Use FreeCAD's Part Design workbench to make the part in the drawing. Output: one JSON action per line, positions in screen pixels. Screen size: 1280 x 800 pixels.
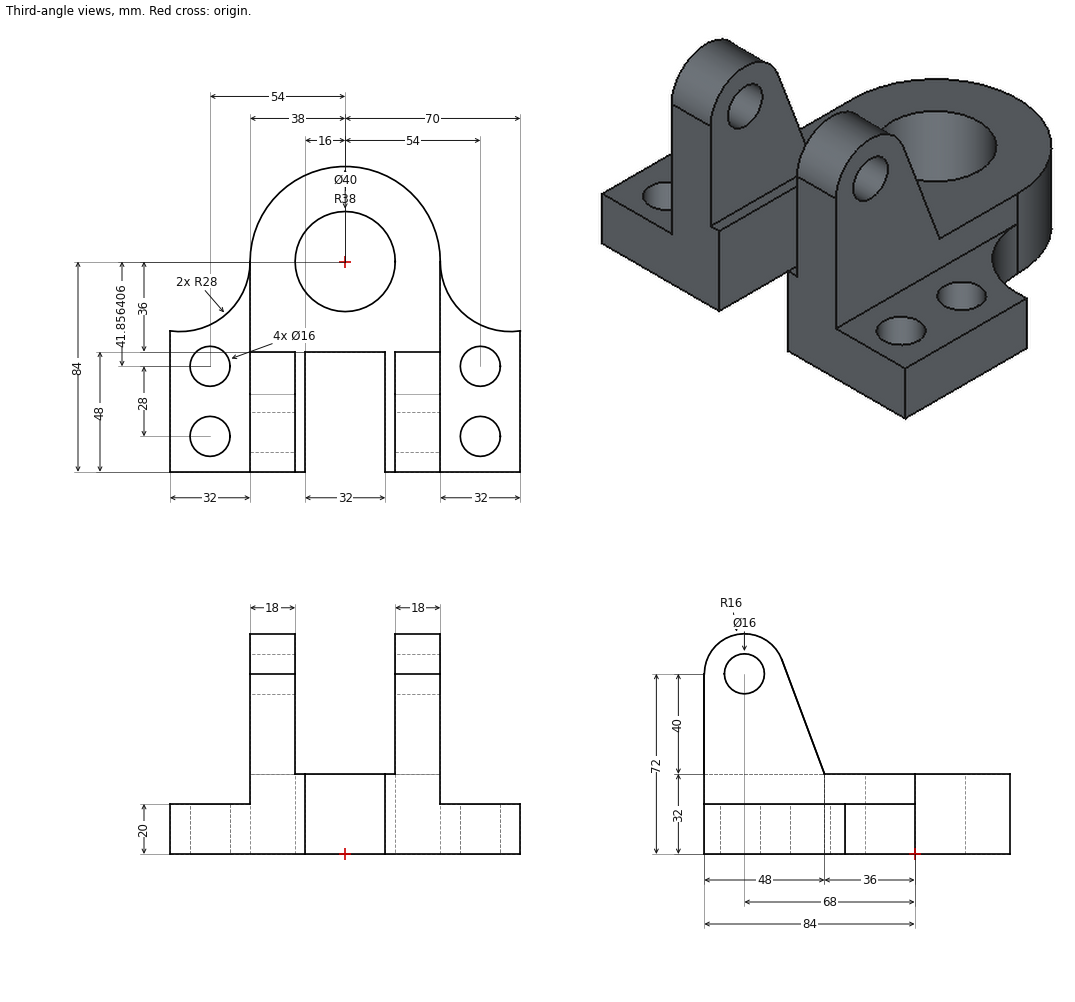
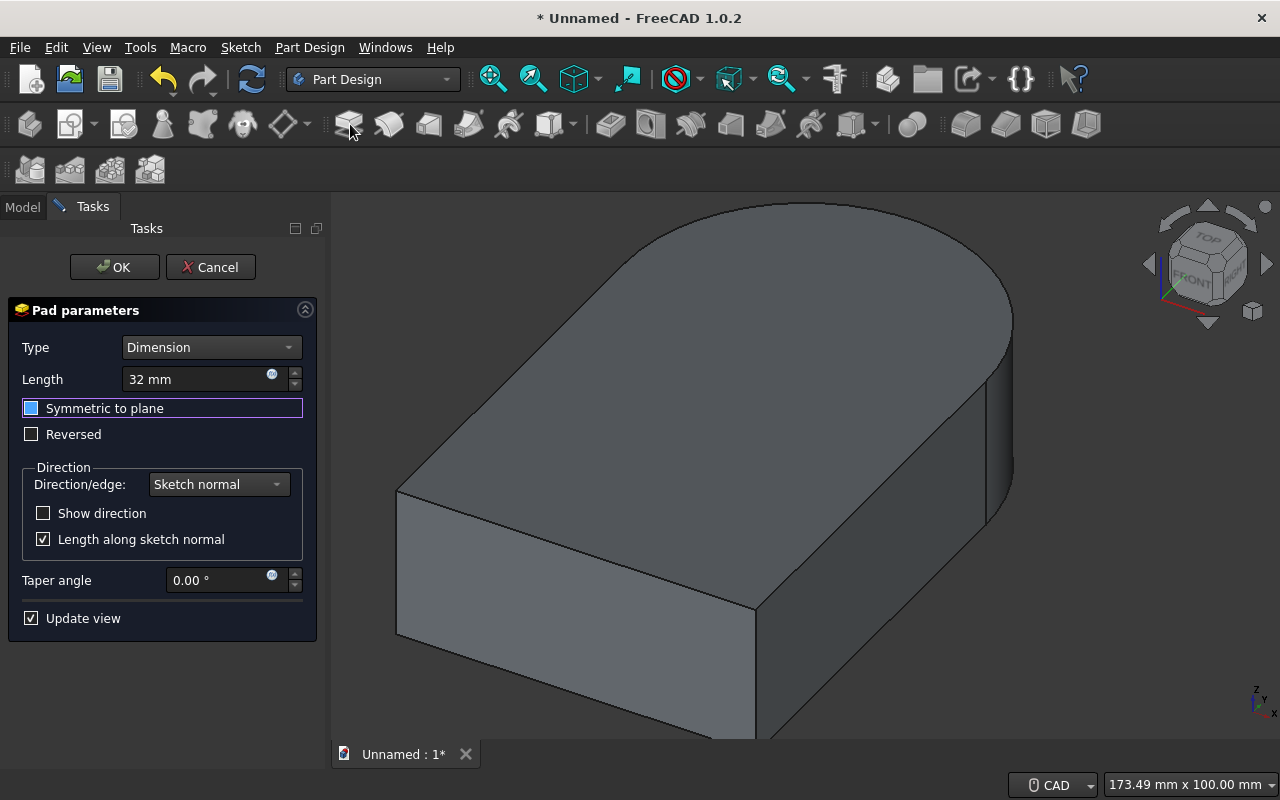
{"action": "left_click", "coordinate": [115, 267]}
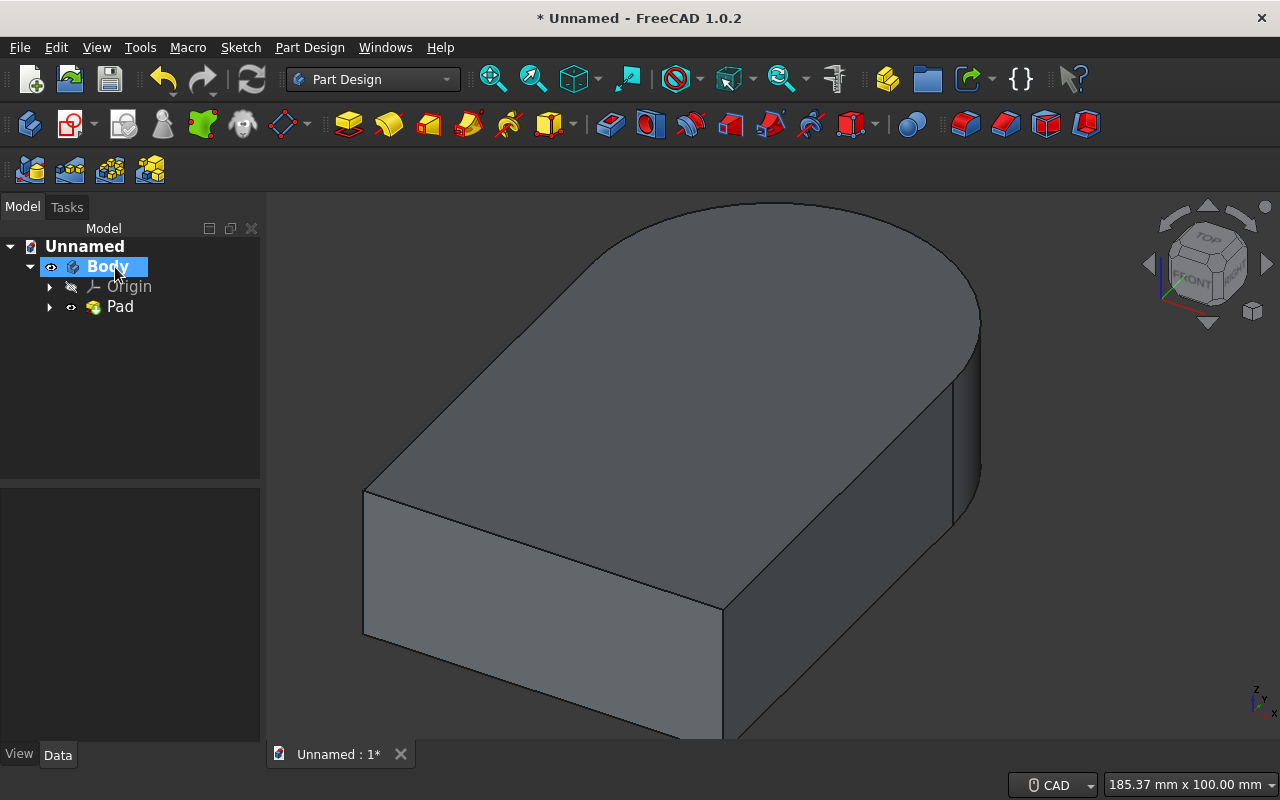
{"action": "left_click", "coordinate": [494, 80]}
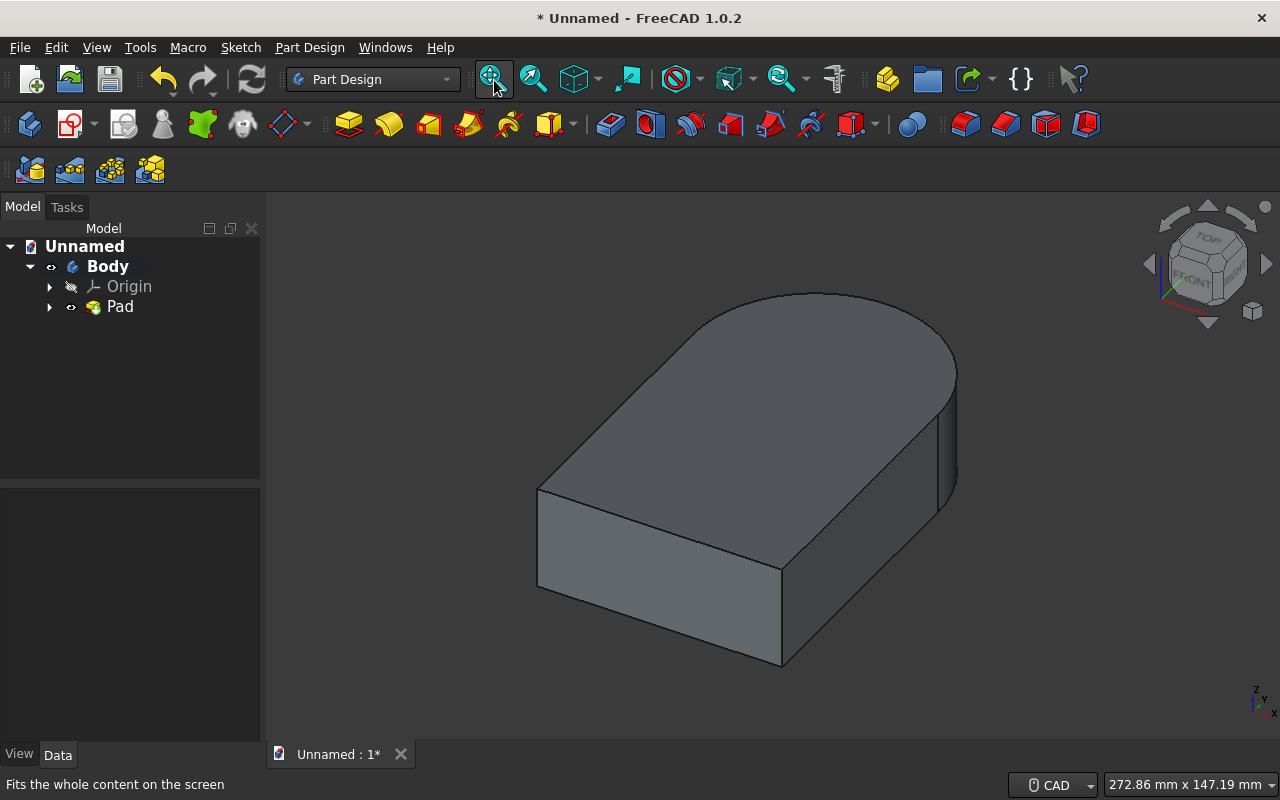
{"action": "left_click", "coordinate": [70, 124]}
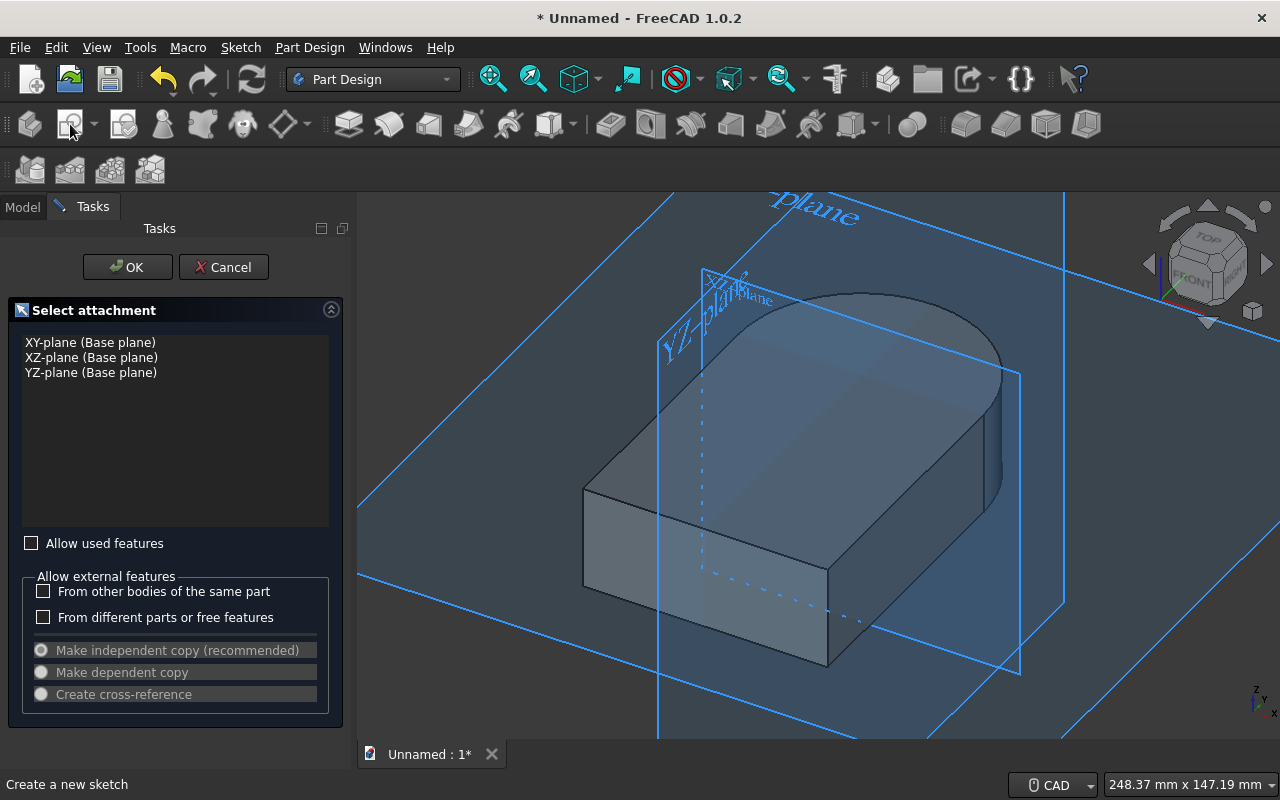
{"action": "left_click", "coordinate": [82, 342]}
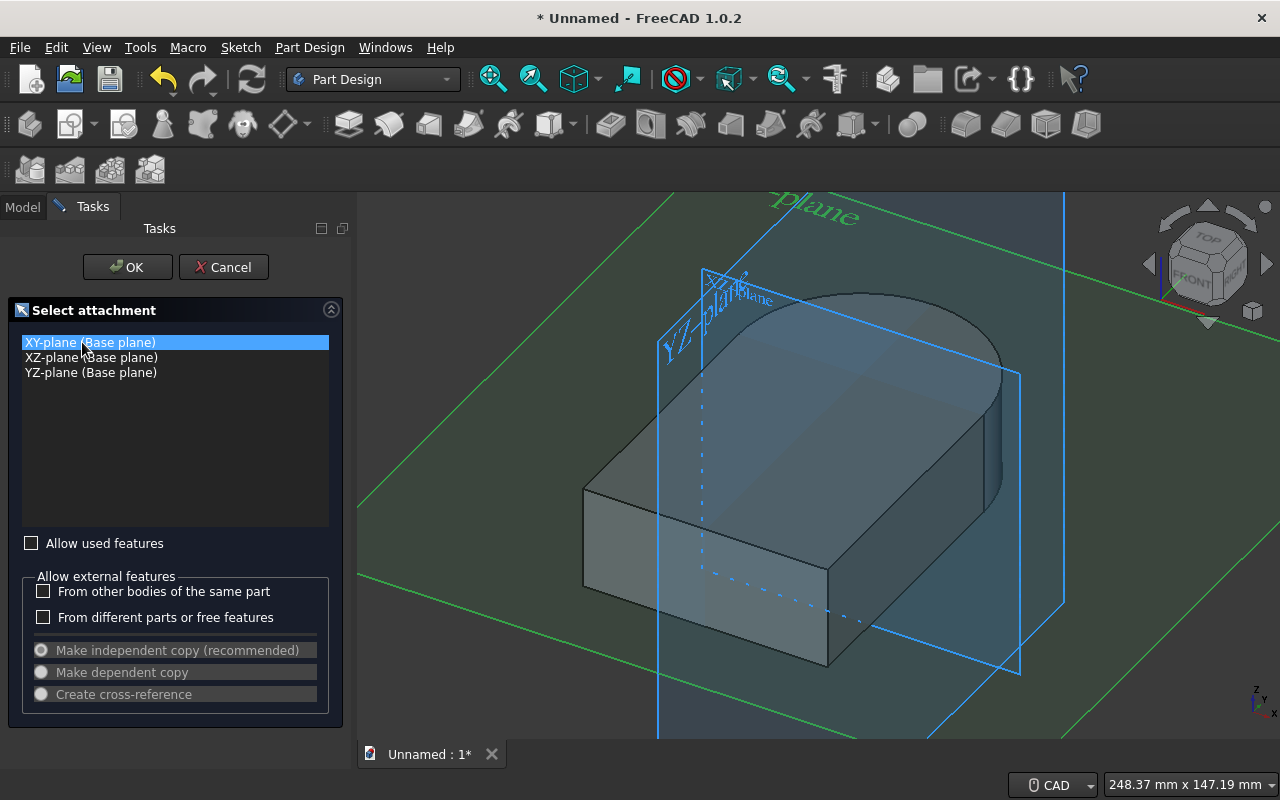
{"action": "left_click", "coordinate": [128, 267]}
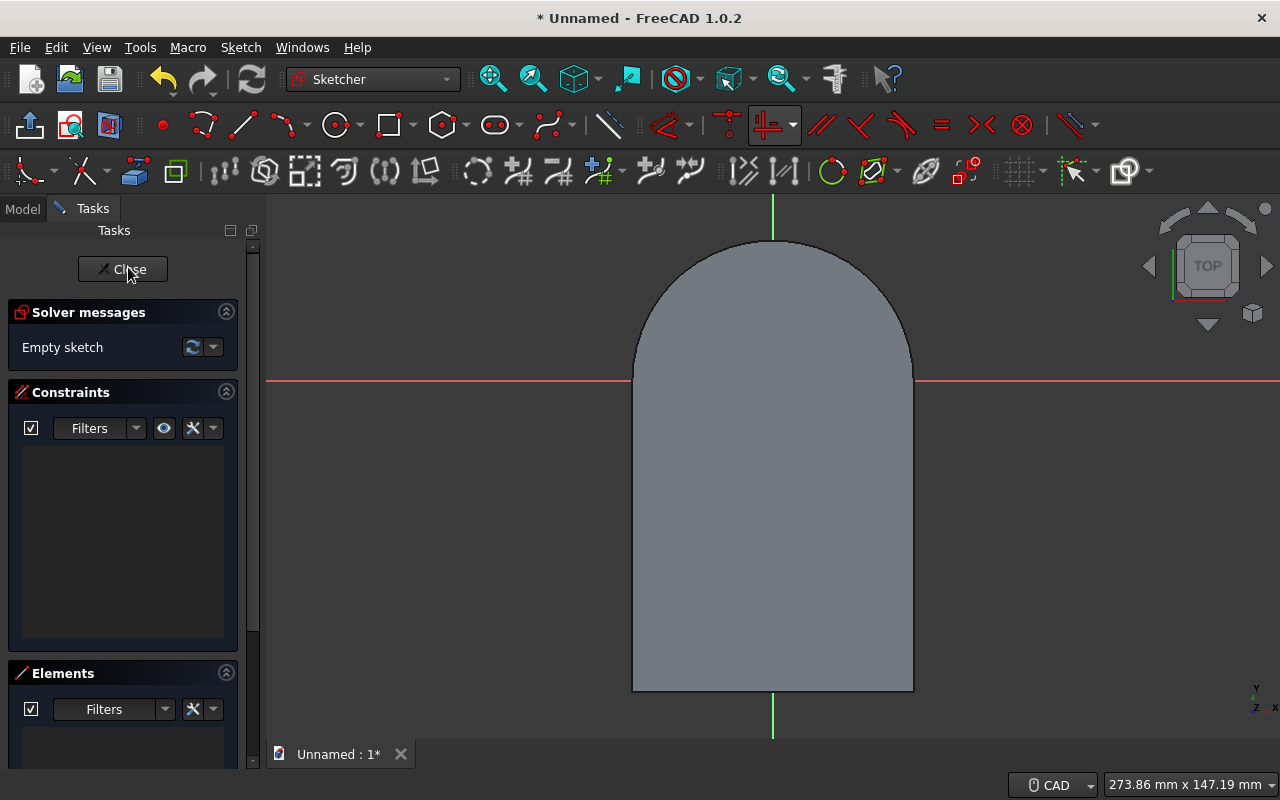
{"action": "left_click", "coordinate": [110, 126]}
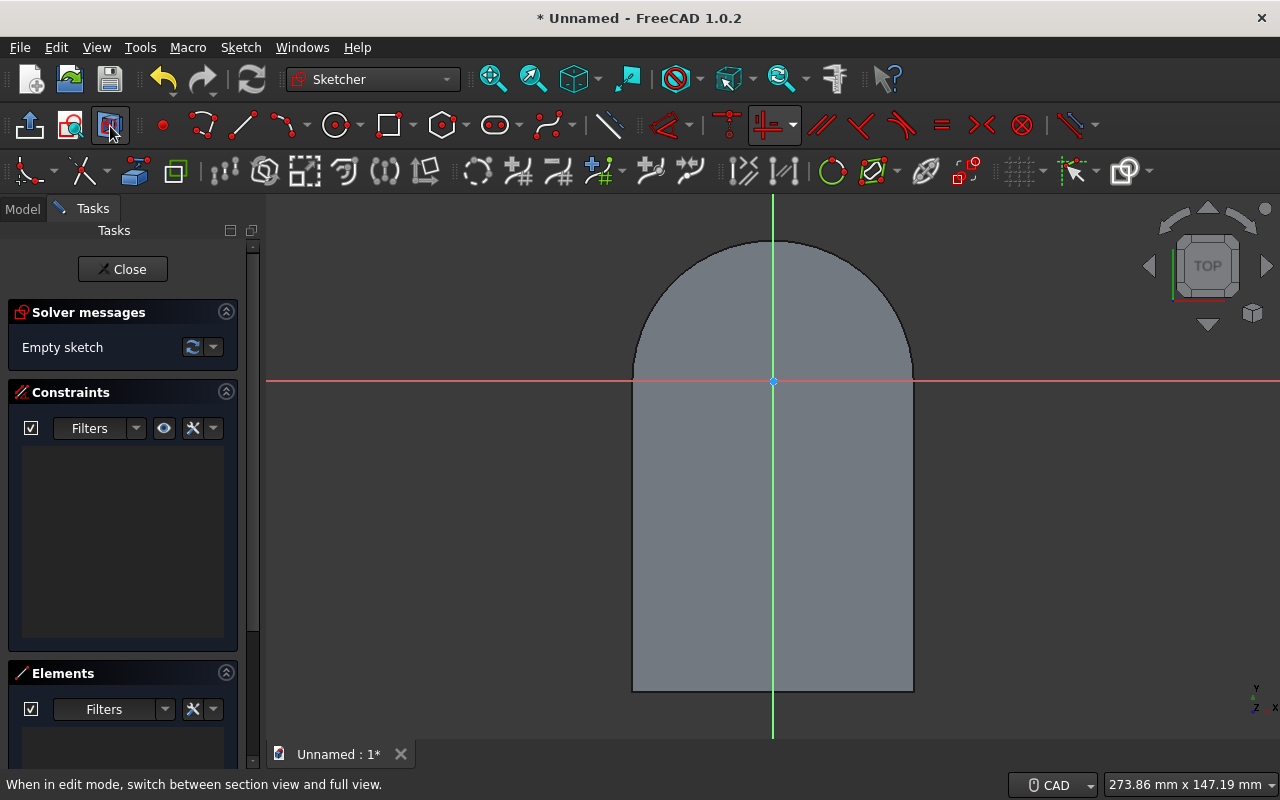
{"action": "scroll", "coordinate": [395, 222], "scroll_direction": "down", "scroll_amount": 1}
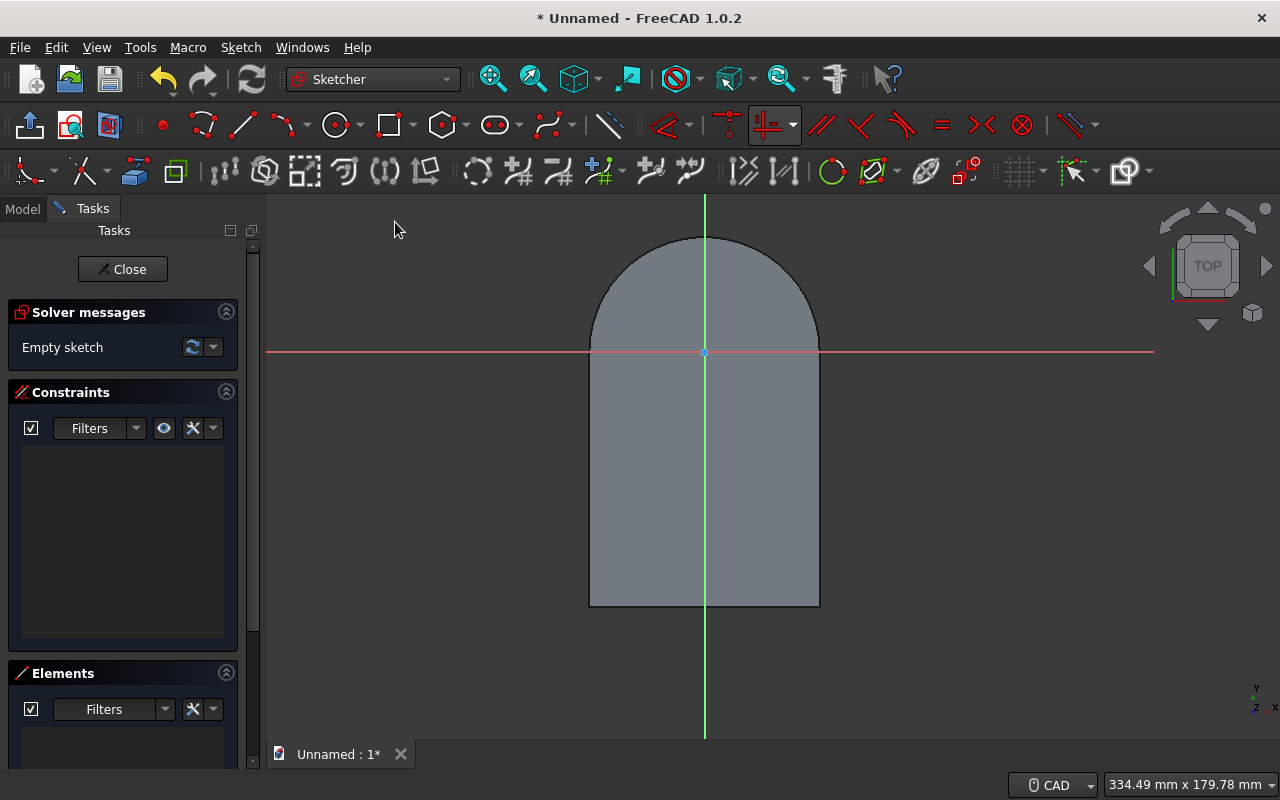
{"action": "scroll", "coordinate": [705, 506], "scroll_direction": "up", "scroll_amount": 2}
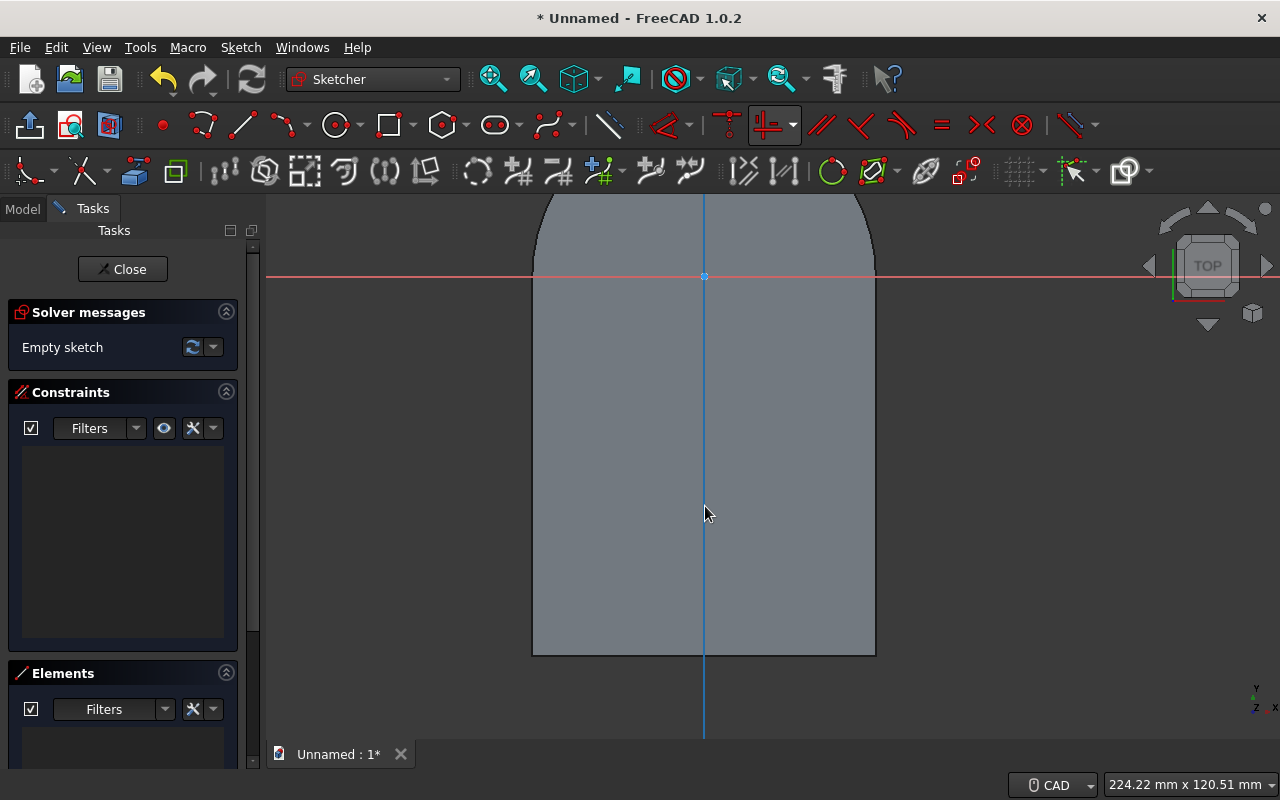
{"action": "left_click", "coordinate": [204, 126]}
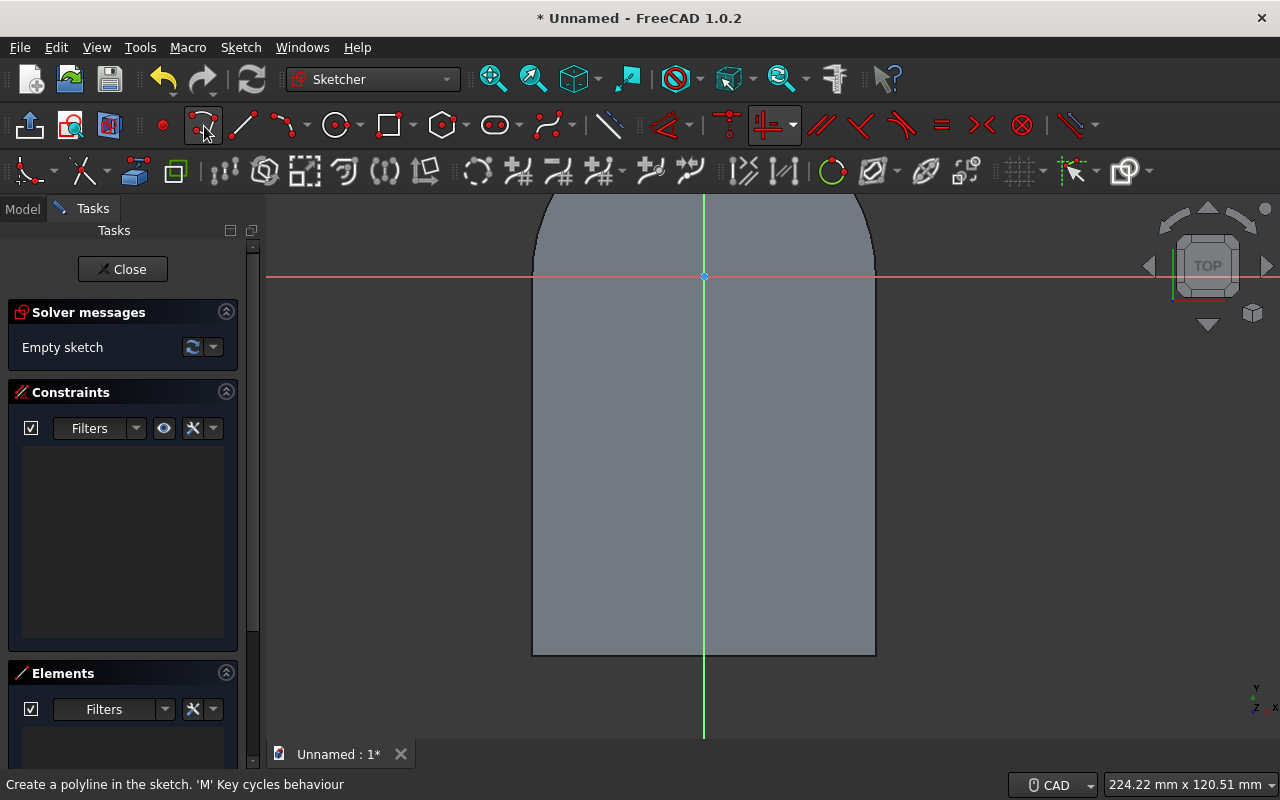
{"action": "left_click", "coordinate": [532, 277]}
{"action": "left_click", "coordinate": [532, 656]}
{"action": "left_click", "coordinate": [387, 656]}
{"action": "left_click", "coordinate": [387, 402]}
{"action": "right_click", "coordinate": [387, 402]}